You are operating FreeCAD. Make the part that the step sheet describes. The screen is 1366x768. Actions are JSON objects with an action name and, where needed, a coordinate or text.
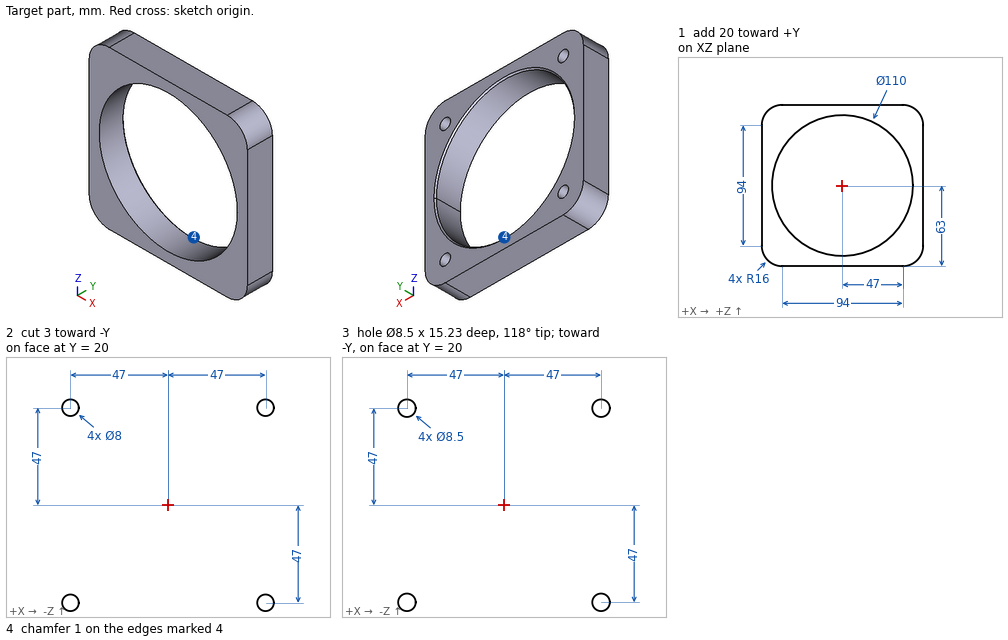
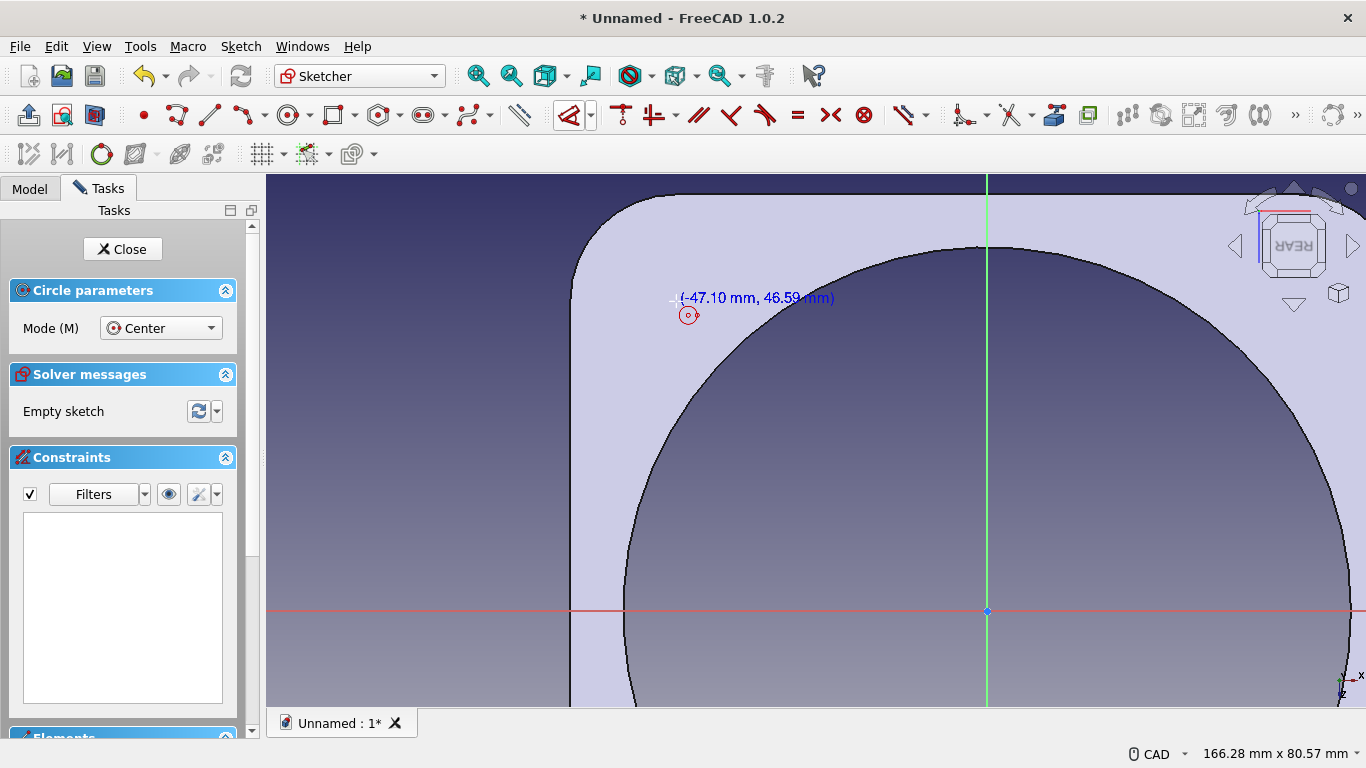
{"action": "left_click", "coordinate": [676, 300]}
{"action": "left_click", "coordinate": [695, 282]}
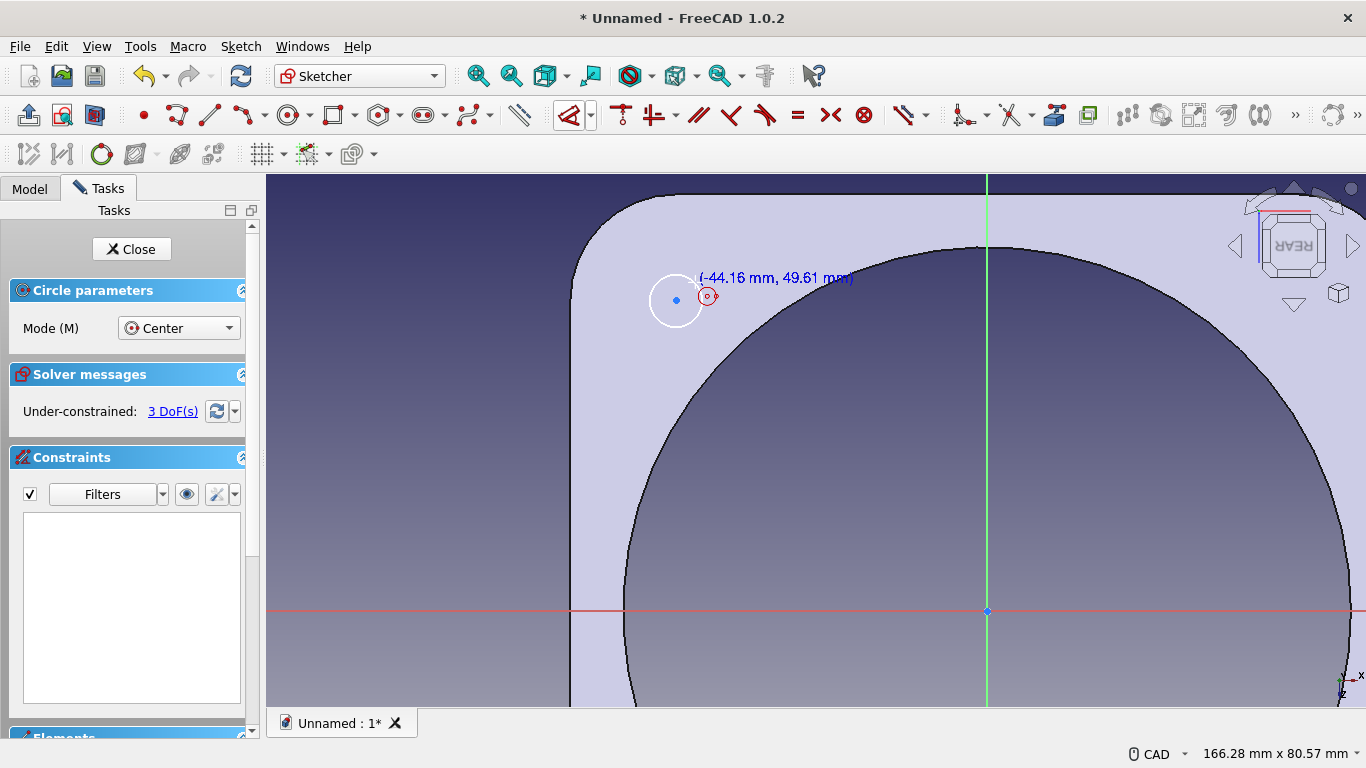
{"action": "scroll", "coordinate": [456, 233], "scroll_direction": "down", "scroll_amount": 3}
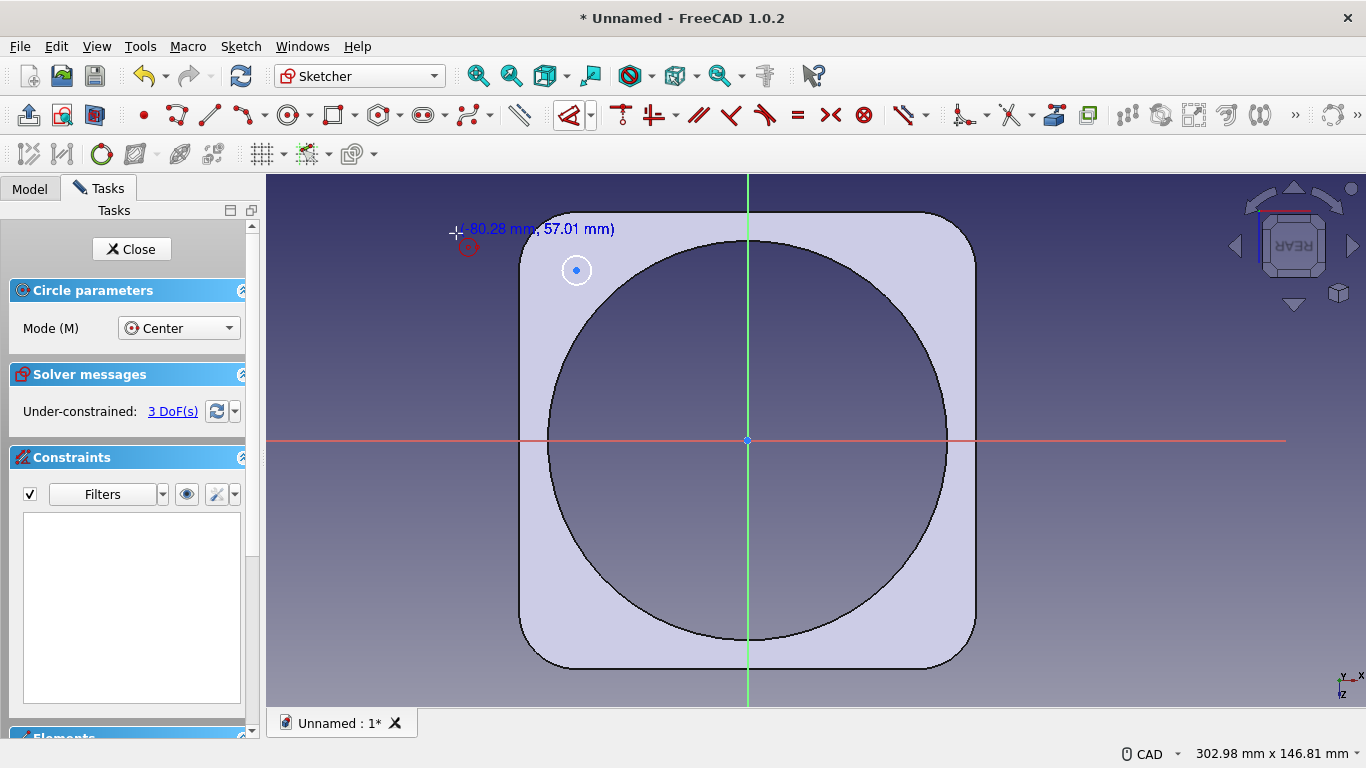
{"action": "scroll", "coordinate": [918, 270], "scroll_direction": "up", "scroll_amount": 3}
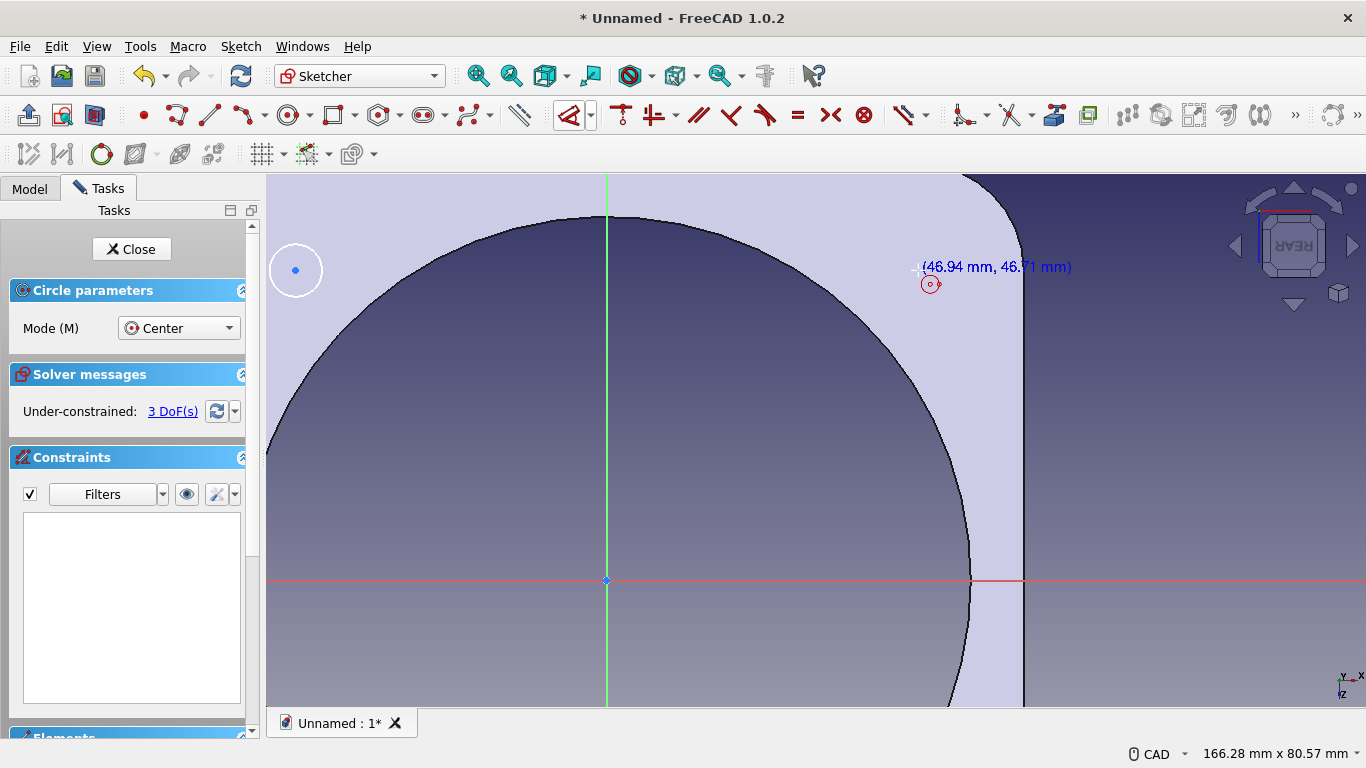
{"action": "left_click", "coordinate": [918, 270]}
{"action": "left_click", "coordinate": [937, 251]}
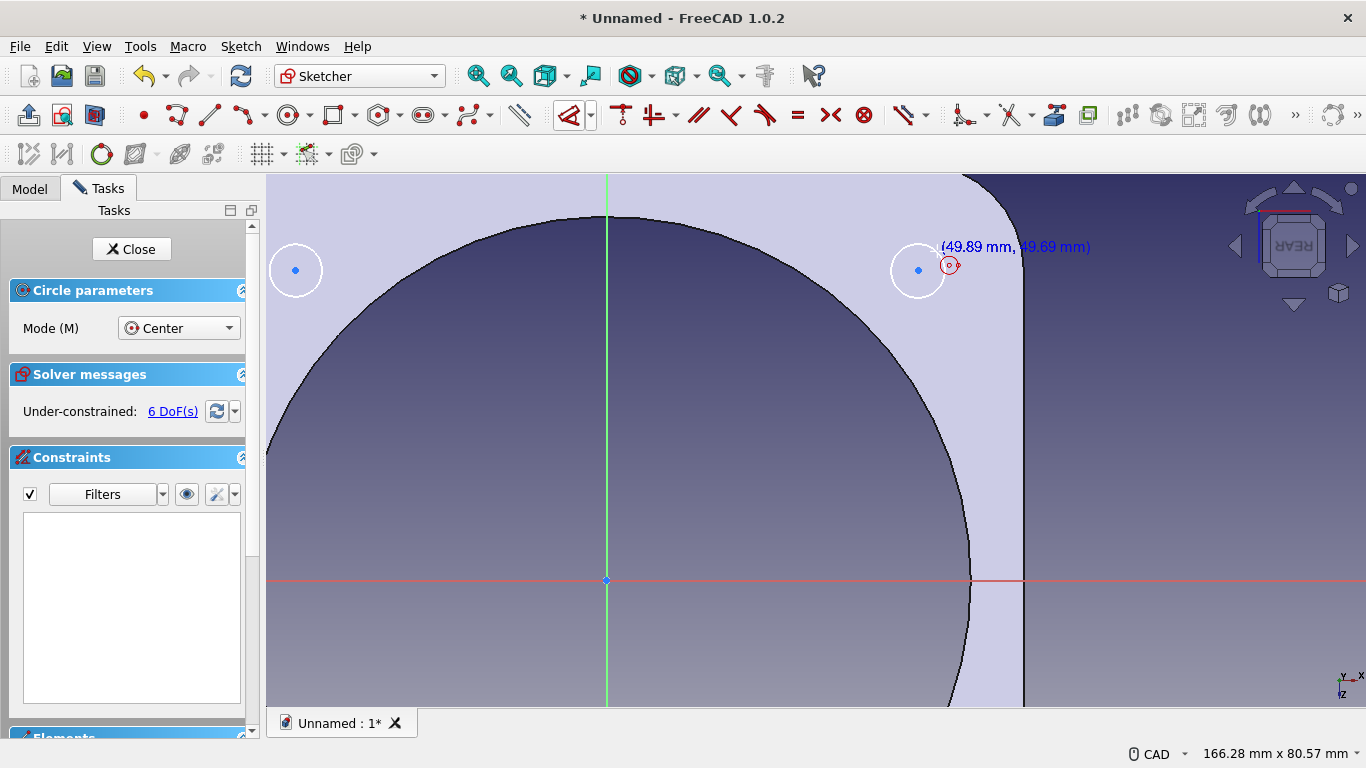
{"action": "scroll", "coordinate": [918, 270], "scroll_direction": "down", "scroll_amount": 3}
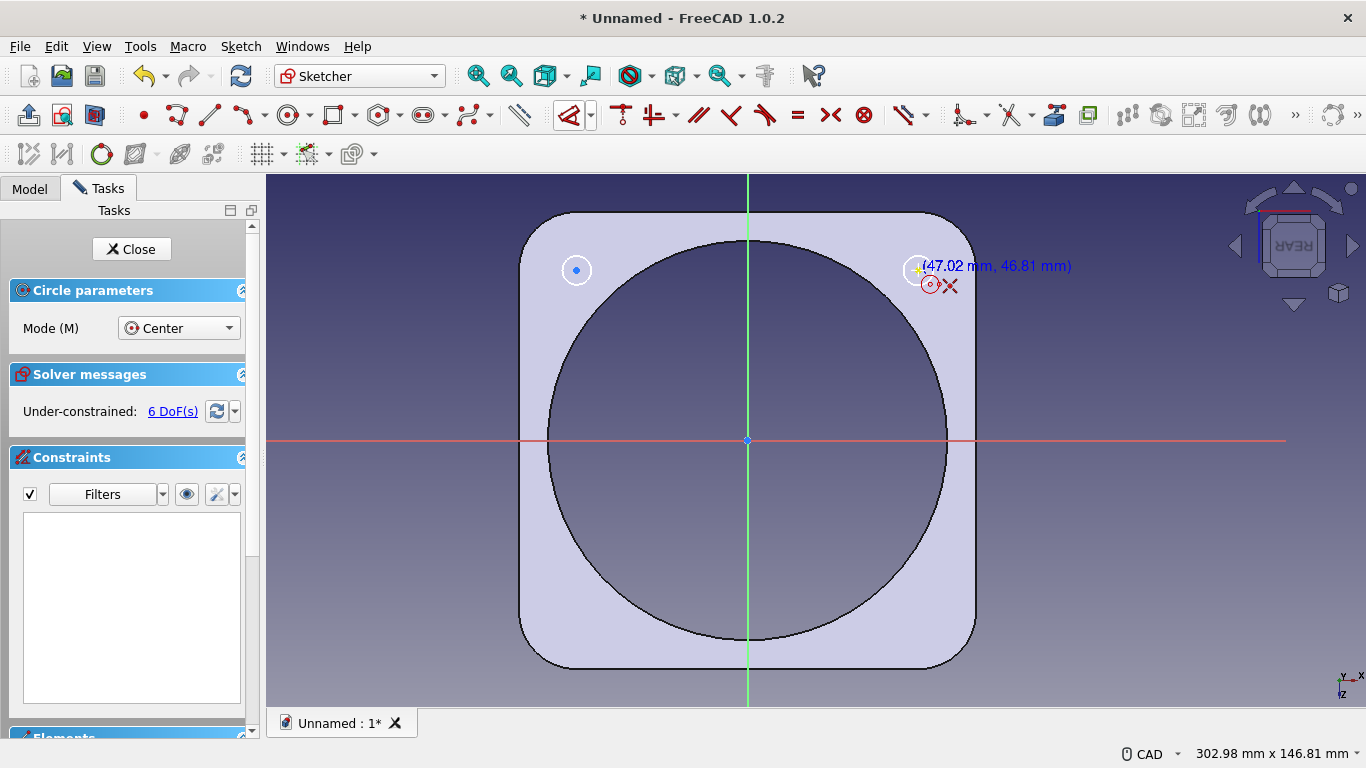
{"action": "scroll", "coordinate": [918, 611], "scroll_direction": "up", "scroll_amount": 3}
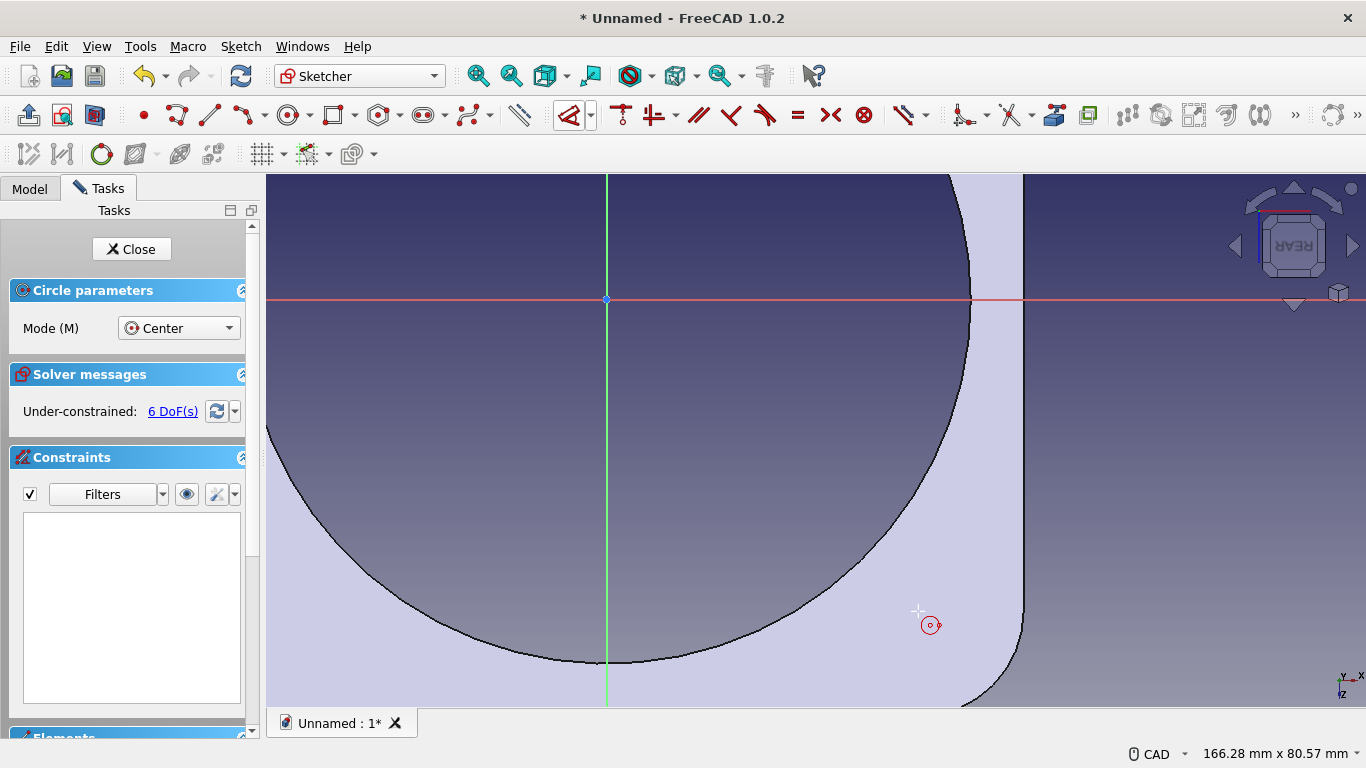
{"action": "left_click", "coordinate": [918, 611]}
{"action": "left_click", "coordinate": [937, 592]}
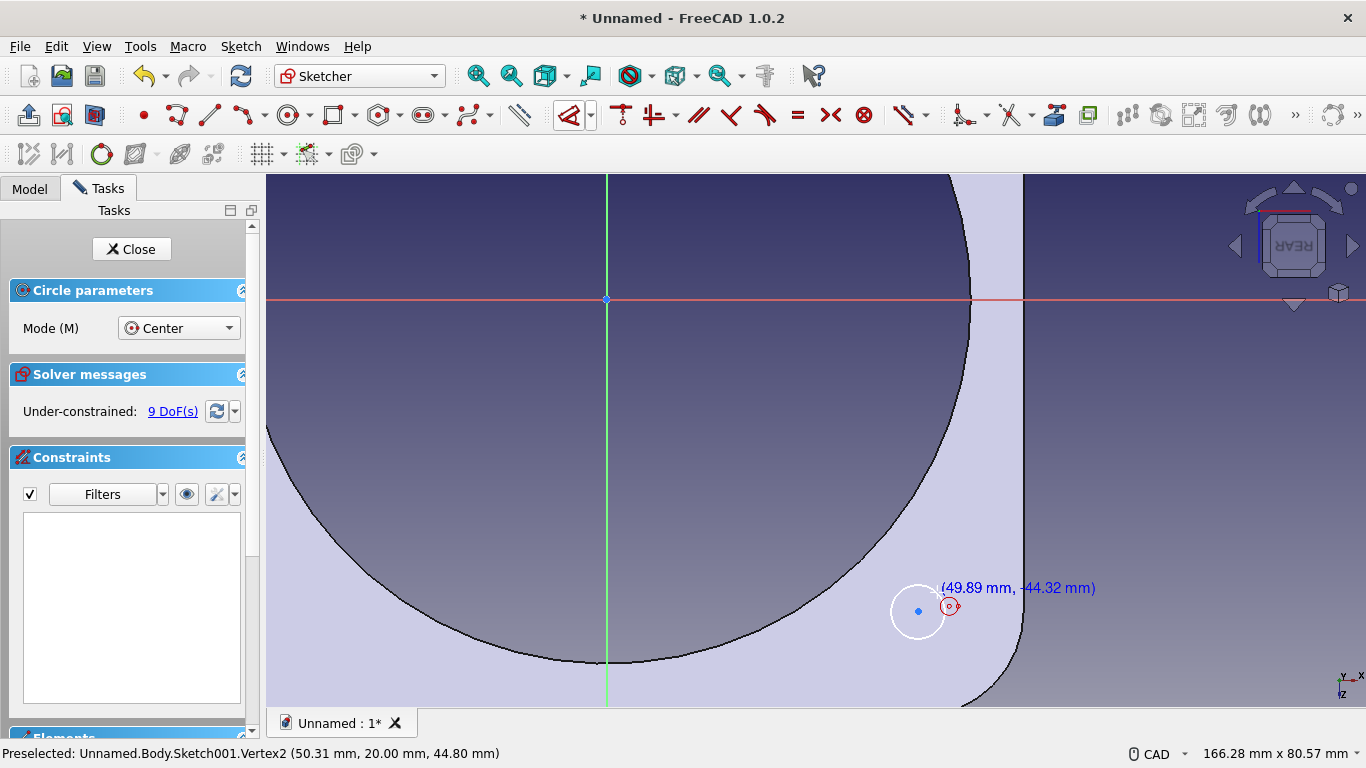
{"action": "left_click", "coordinate": [296, 611]}
{"action": "left_click", "coordinate": [315, 592]}
{"action": "key", "text": "Escape"}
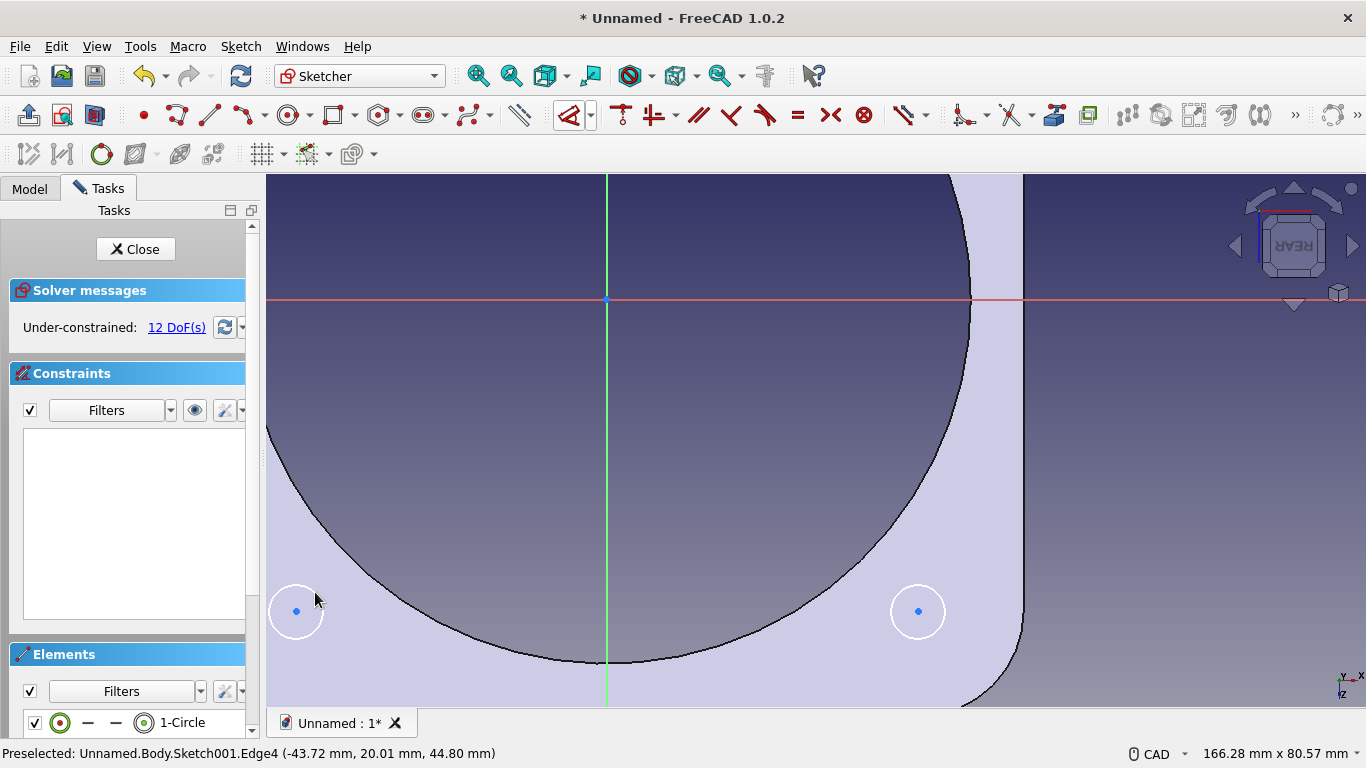
{"action": "scroll", "coordinate": [918, 612], "scroll_direction": "down", "scroll_amount": 3}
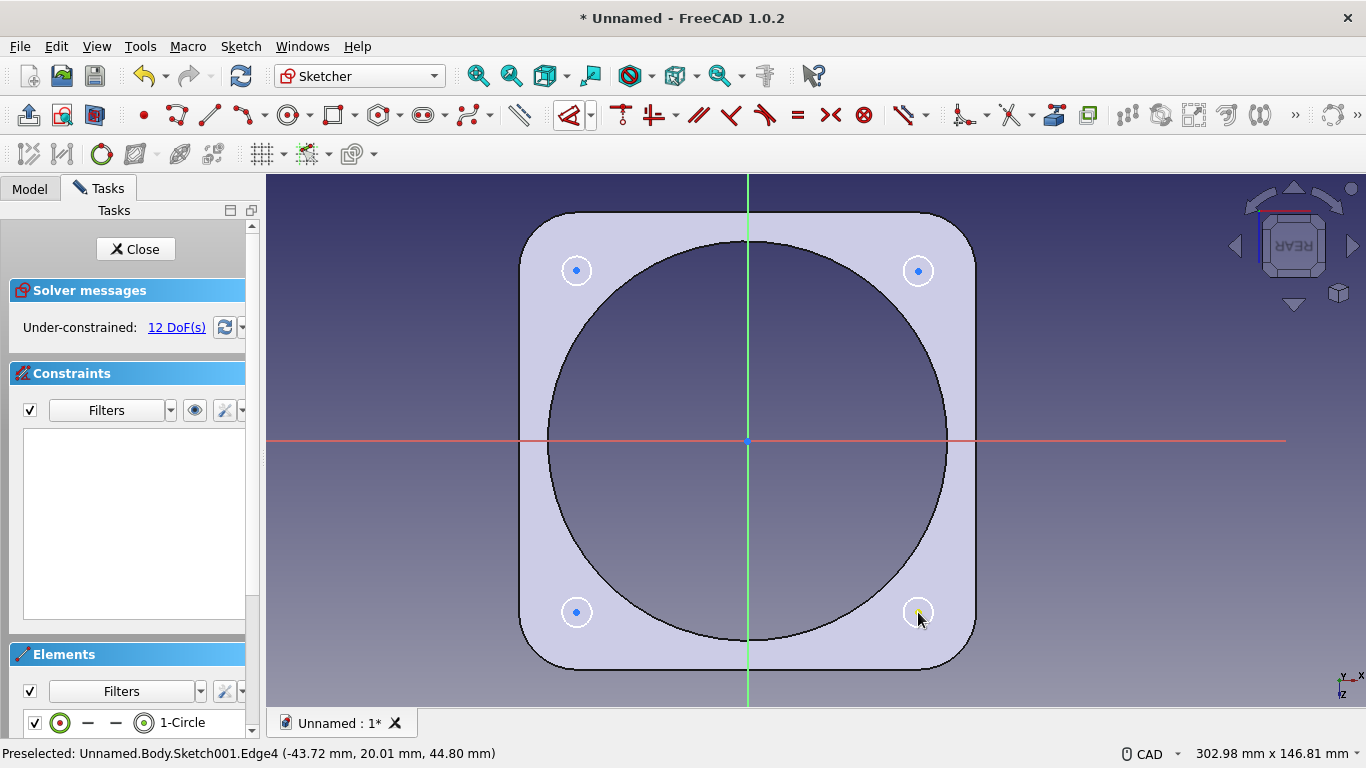
{"action": "left_click", "coordinate": [587, 261]}